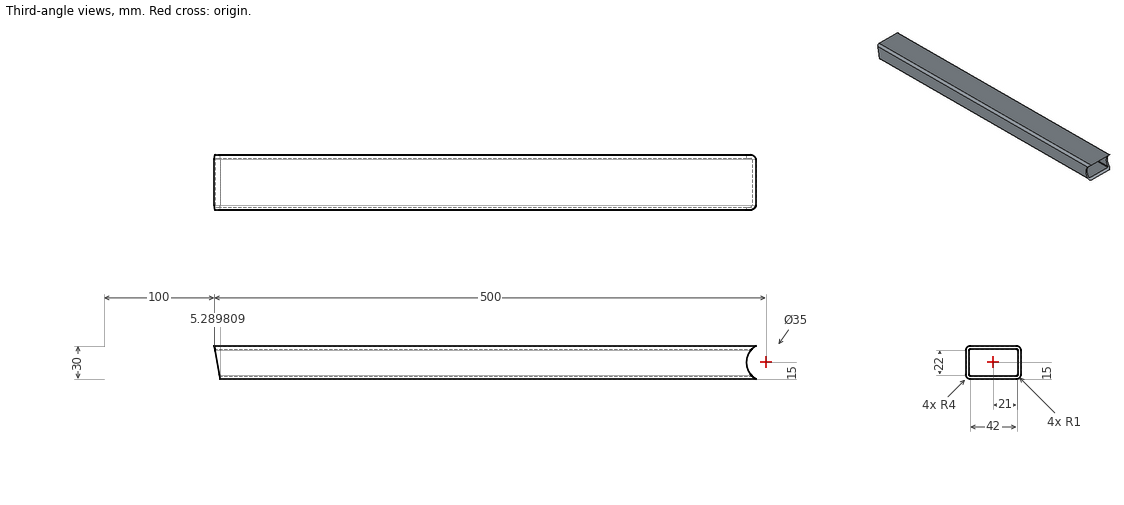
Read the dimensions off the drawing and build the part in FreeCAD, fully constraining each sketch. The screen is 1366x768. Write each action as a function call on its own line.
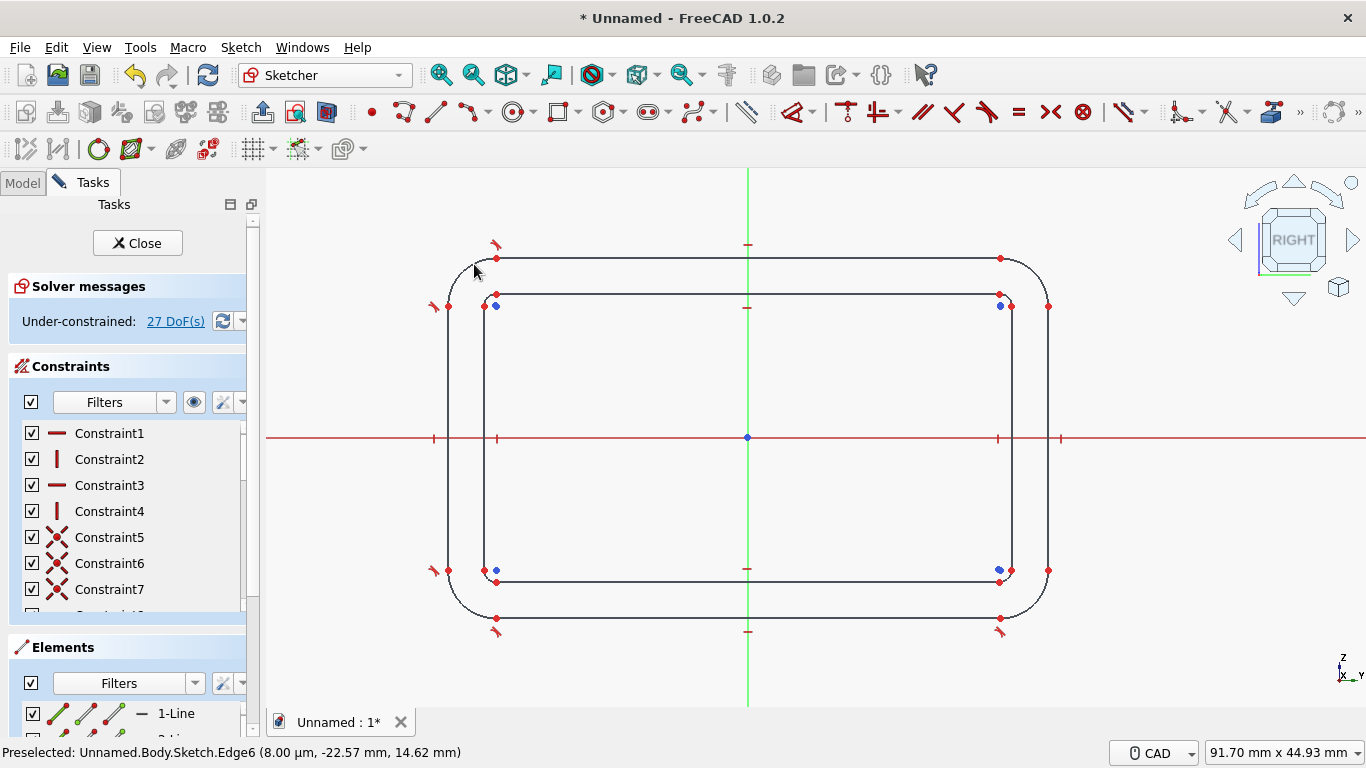
click(647, 258)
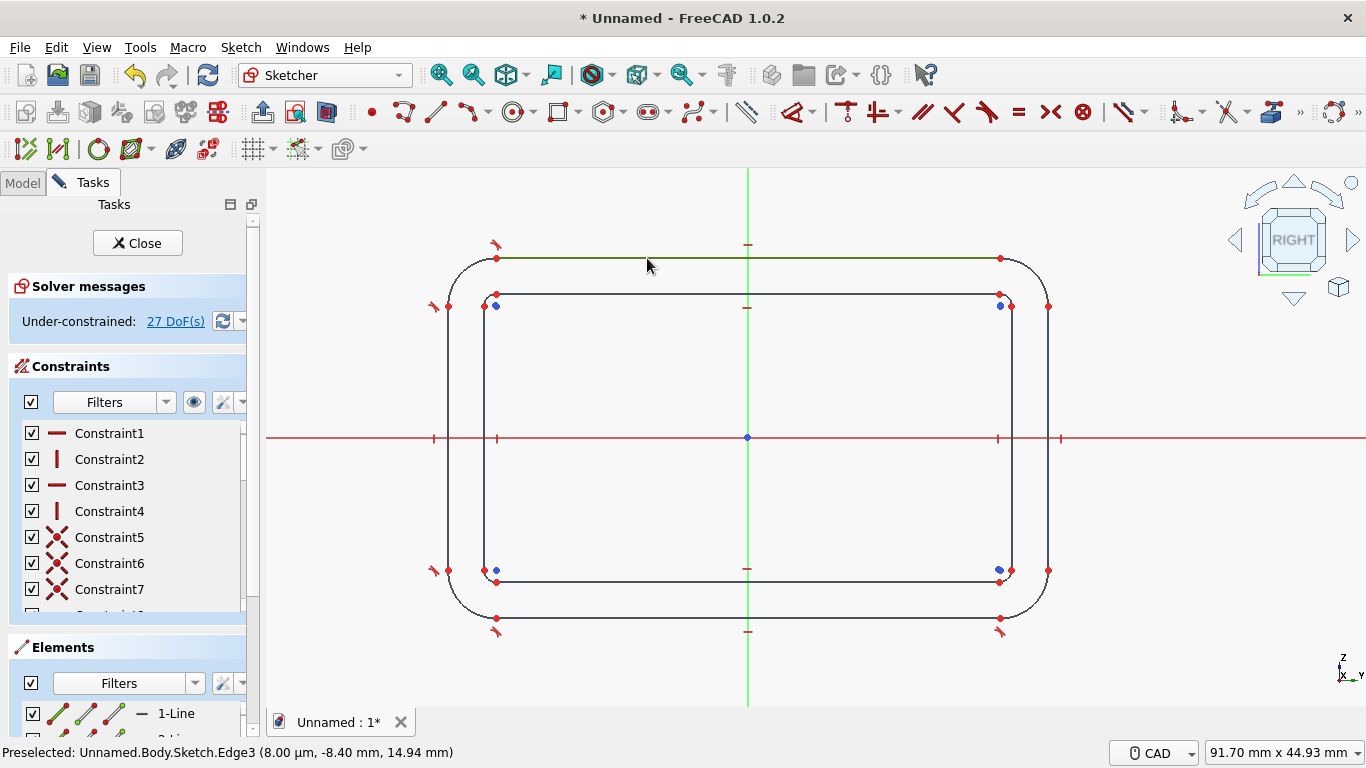
click(1043, 285)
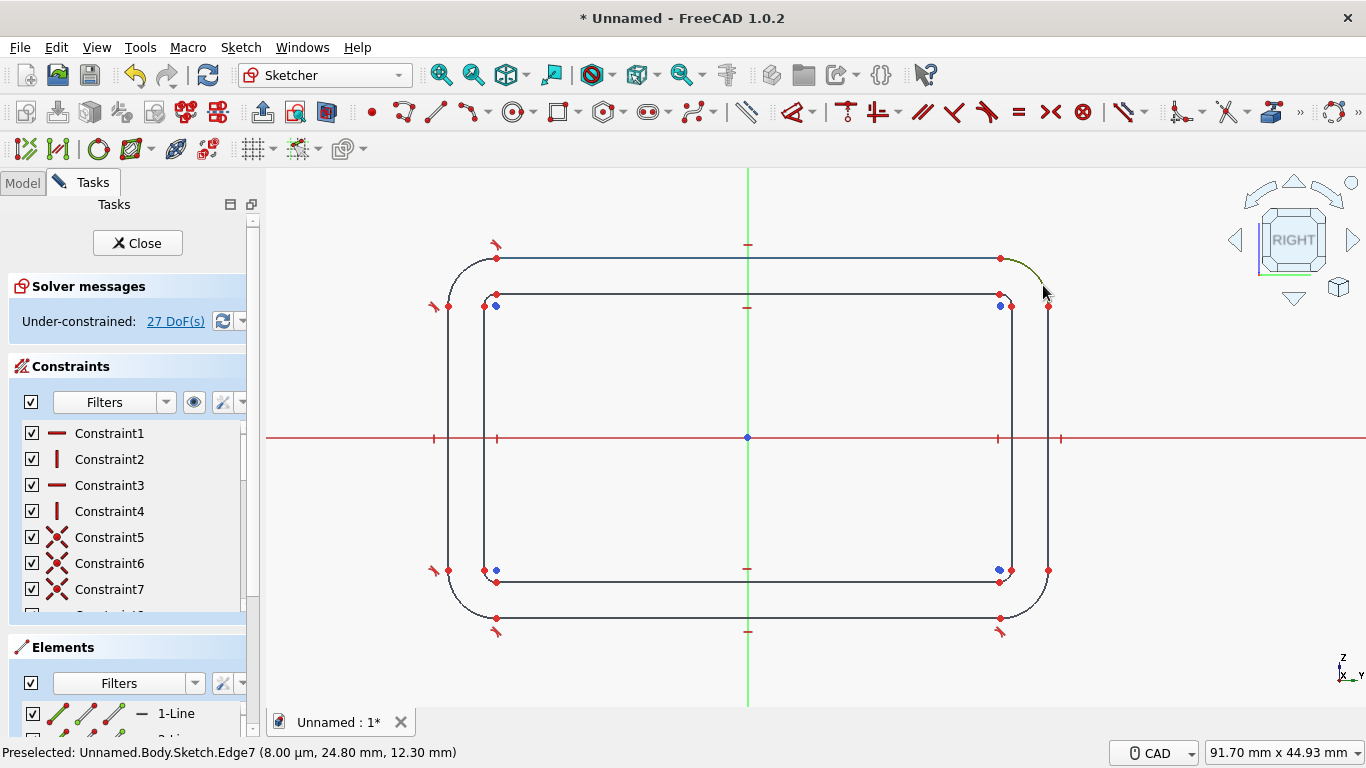
key(t)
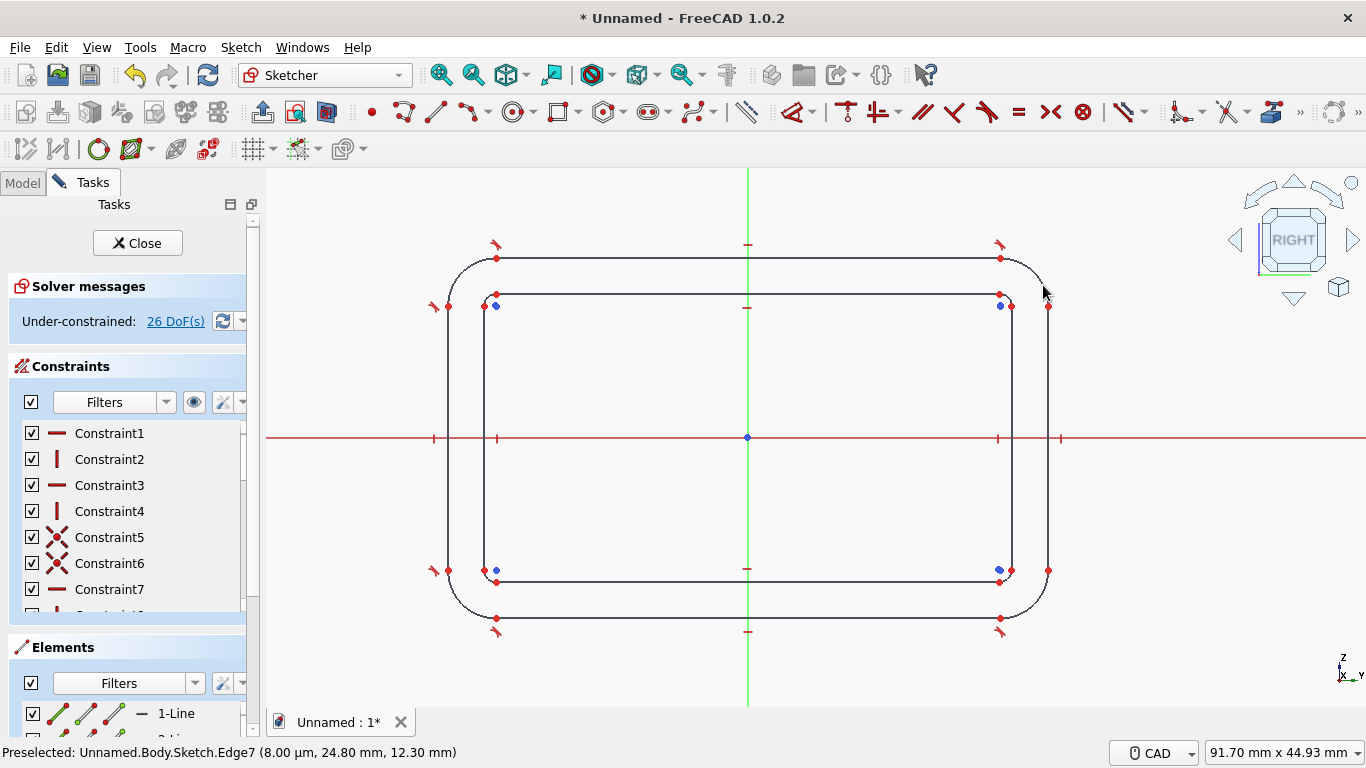
click(1048, 386)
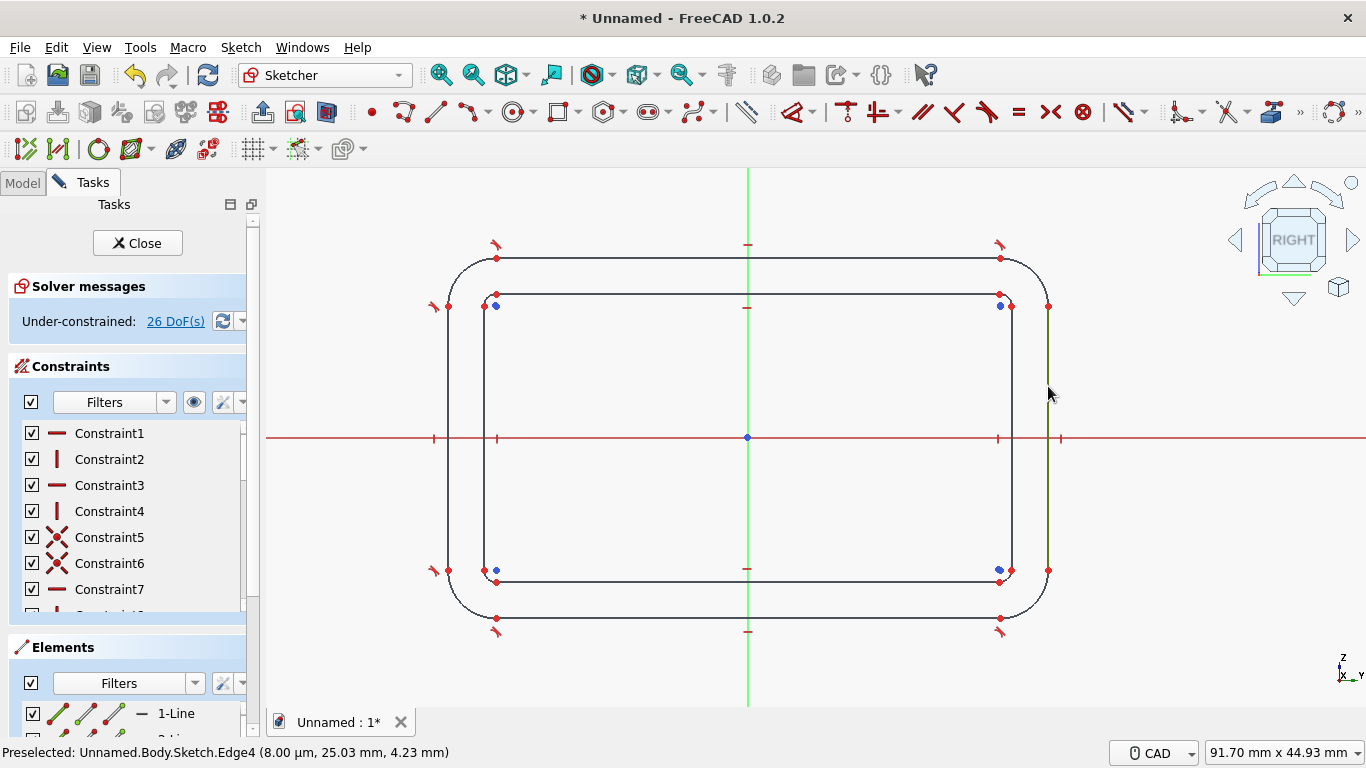
click(1043, 285)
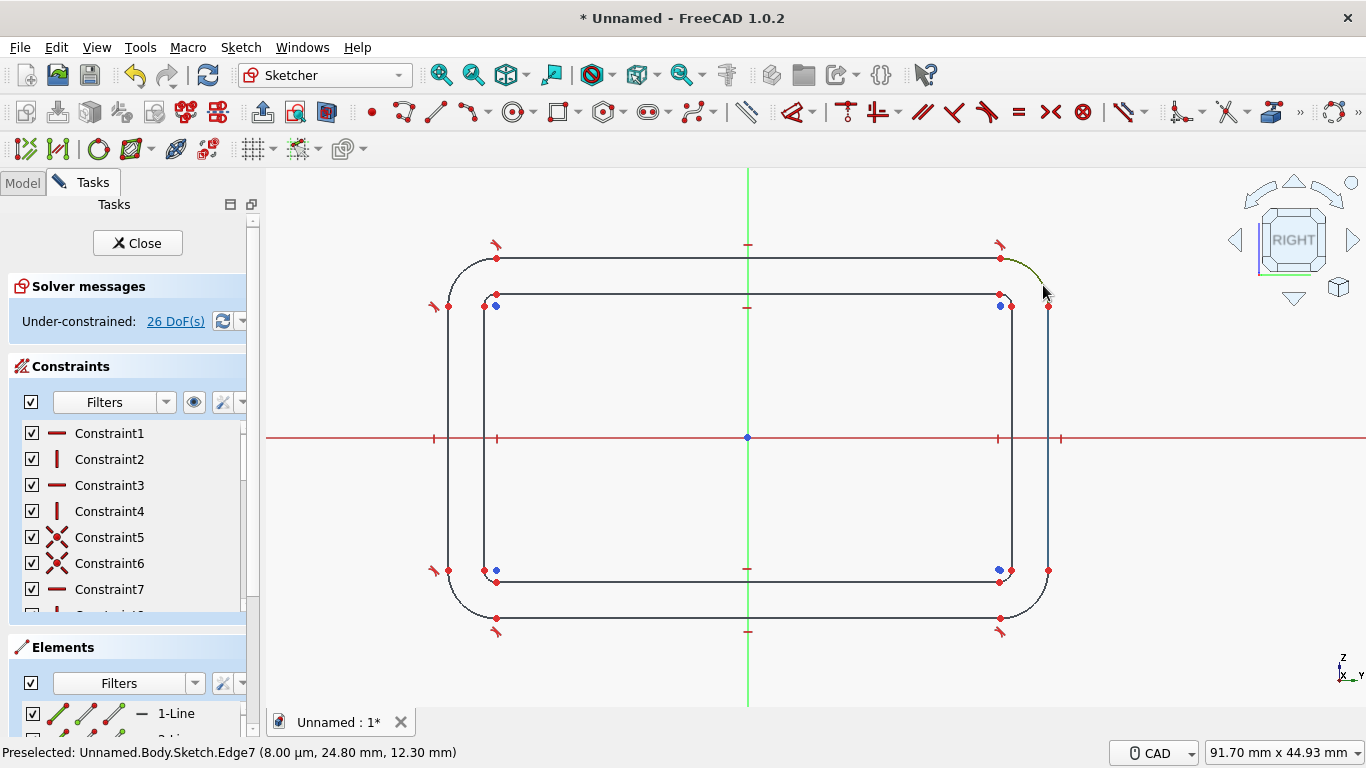
key(t)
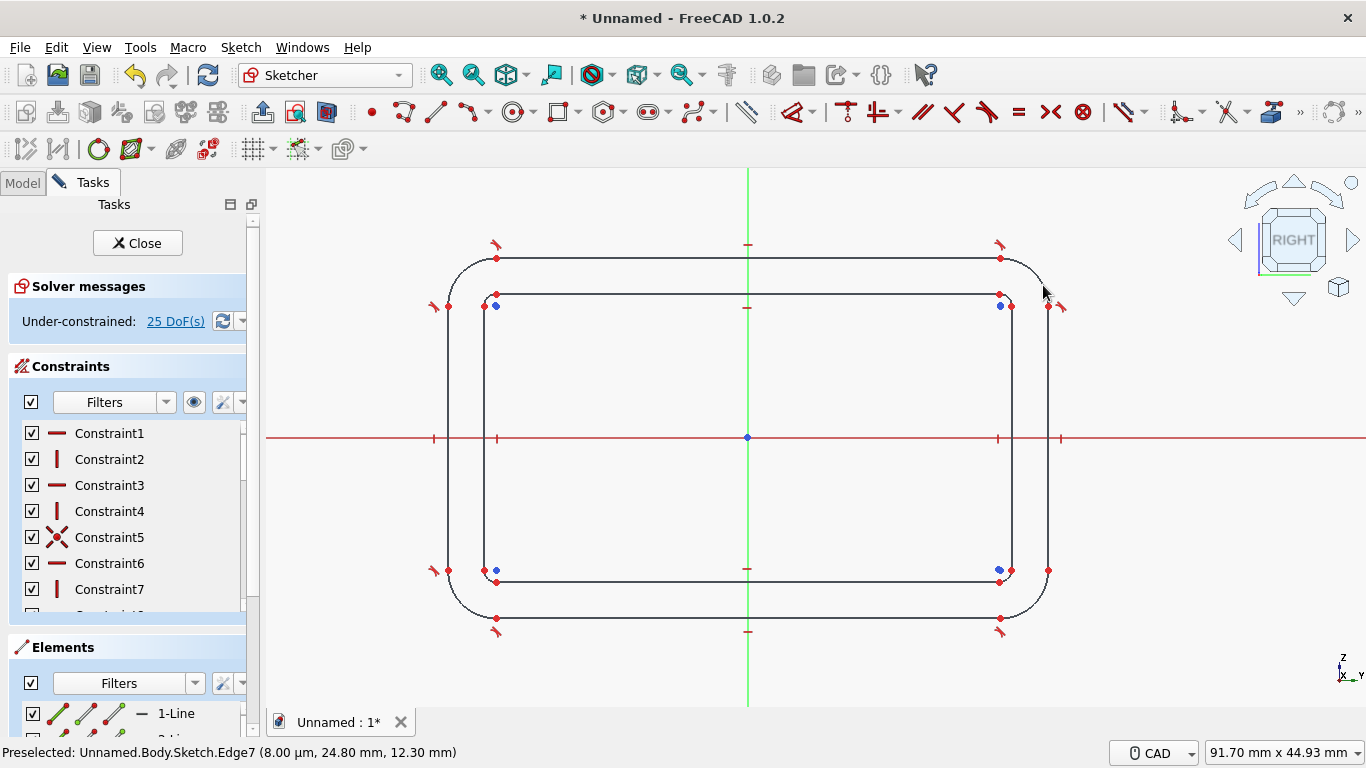
click(1048, 386)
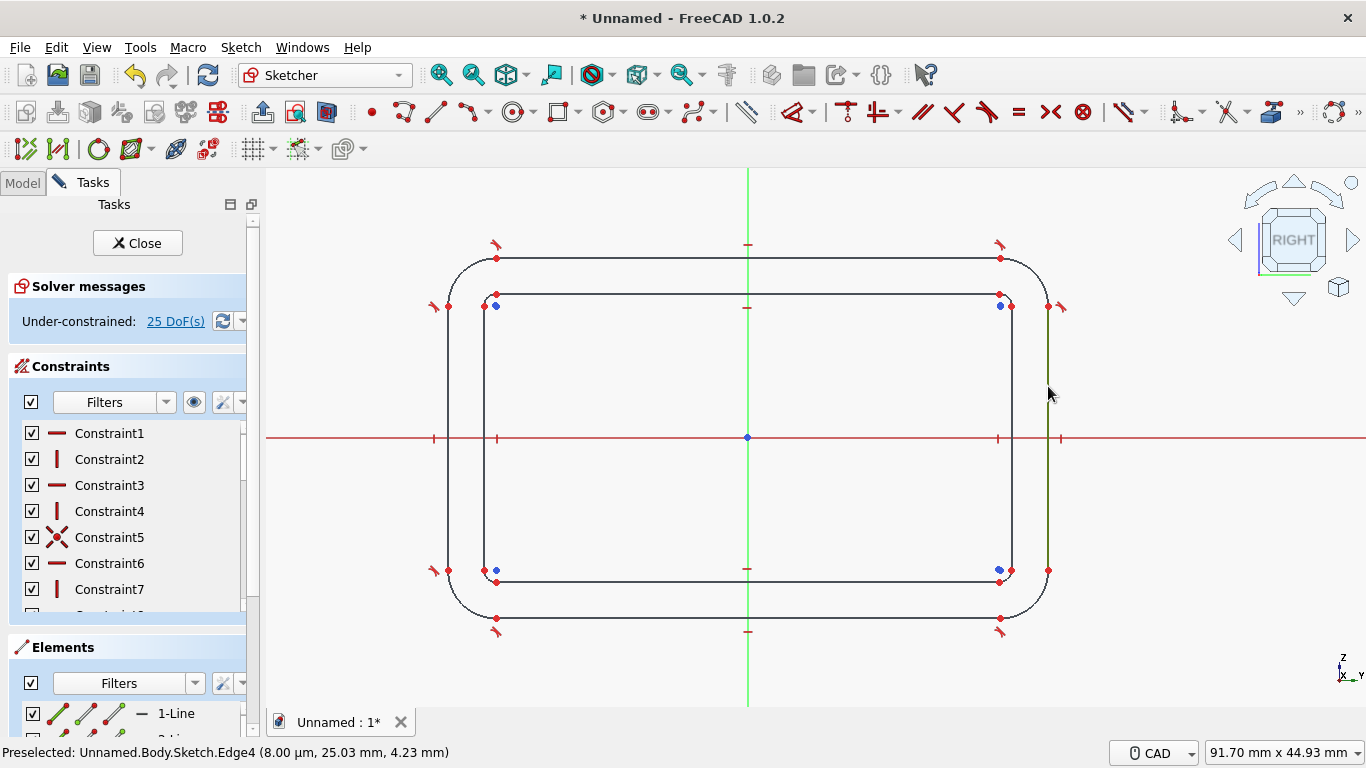
click(1022, 613)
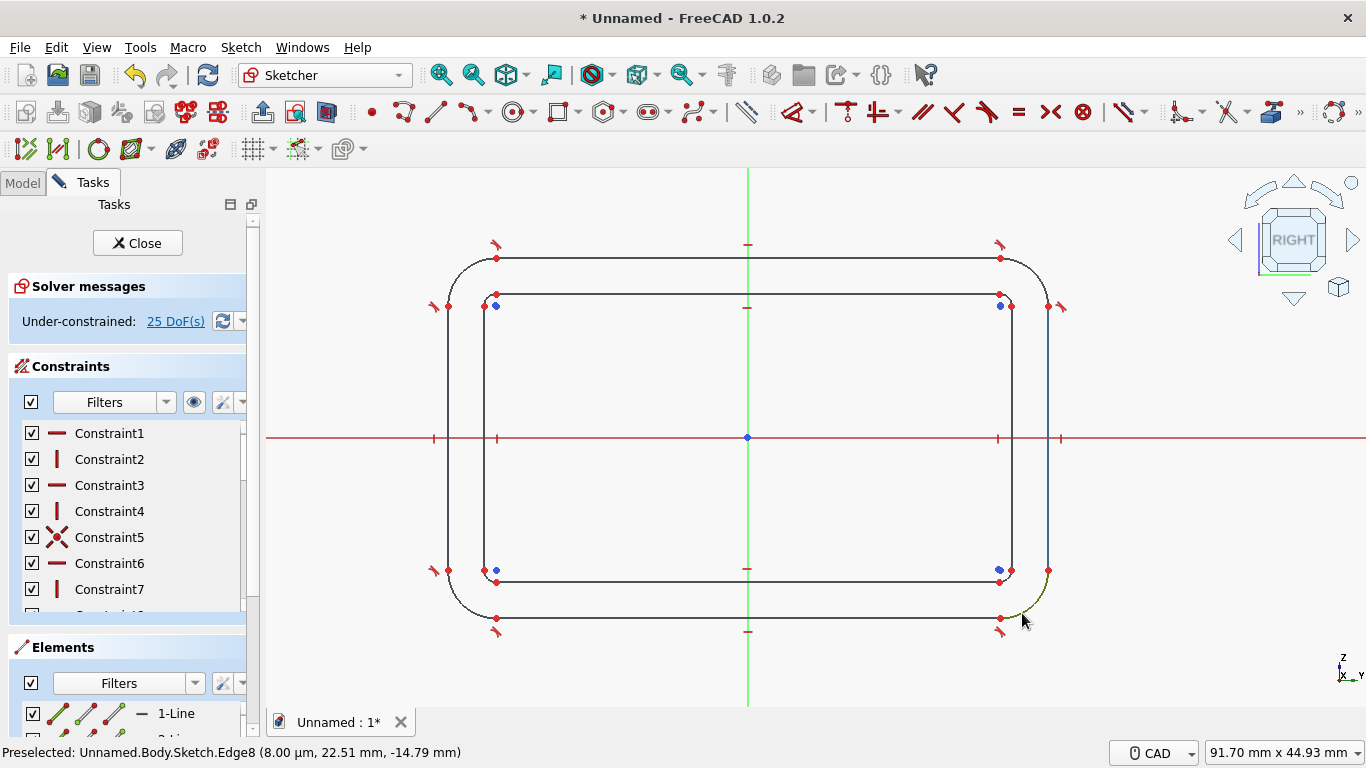
key(t)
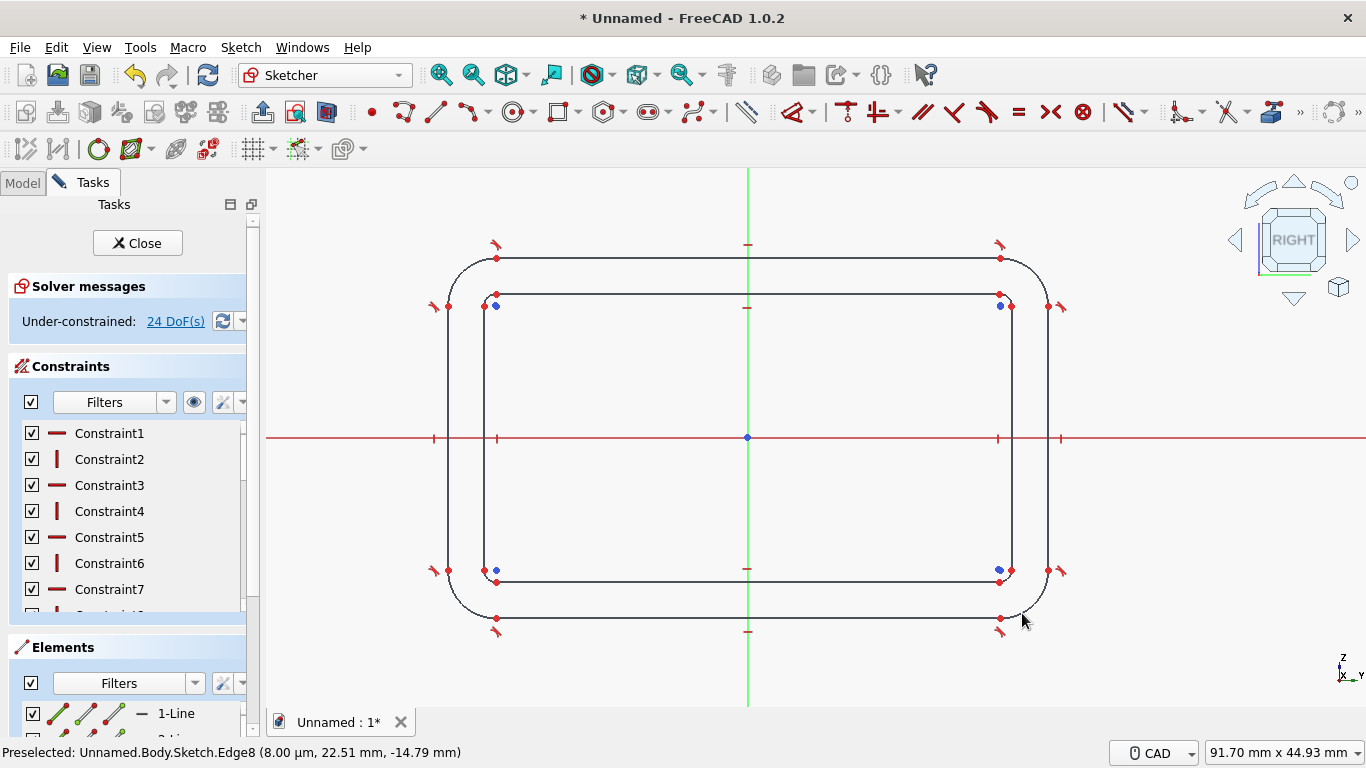
click(647, 582)